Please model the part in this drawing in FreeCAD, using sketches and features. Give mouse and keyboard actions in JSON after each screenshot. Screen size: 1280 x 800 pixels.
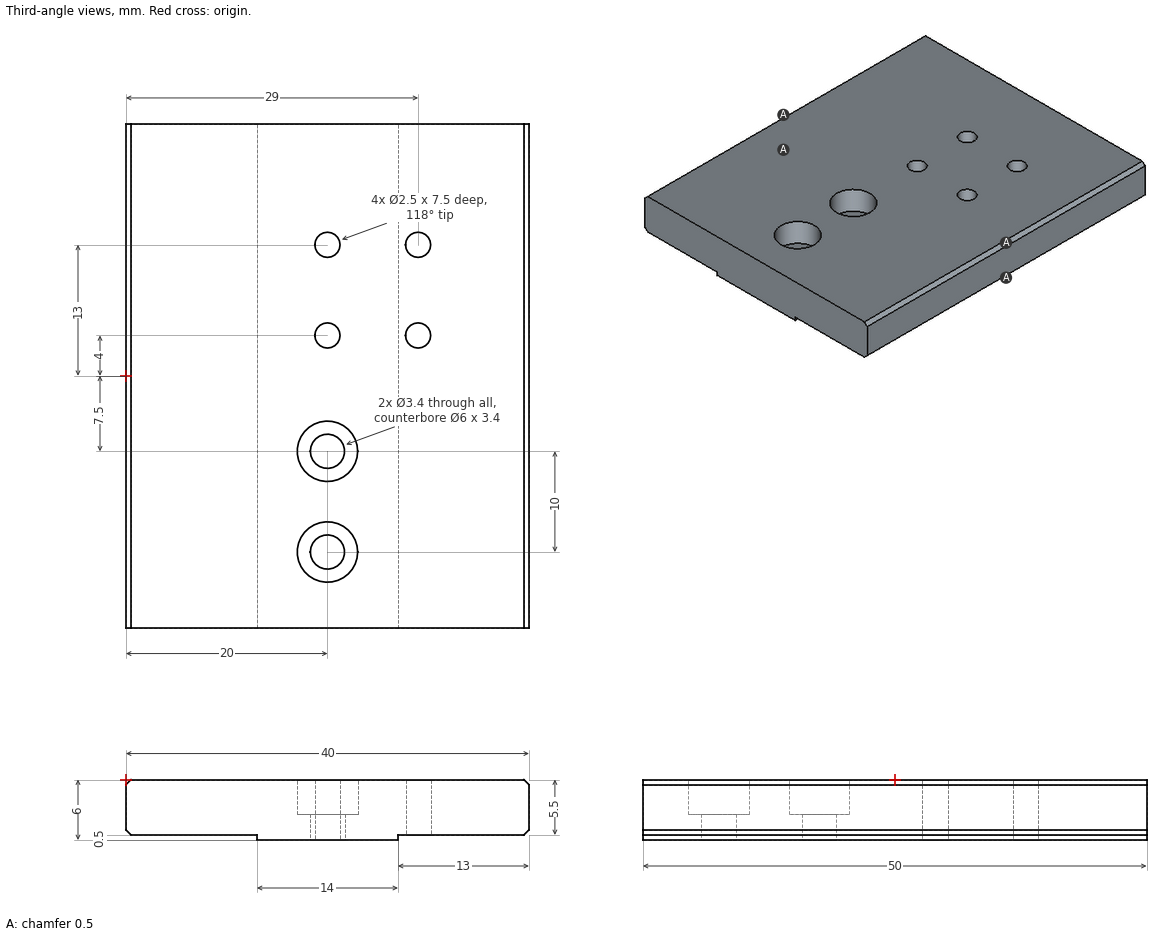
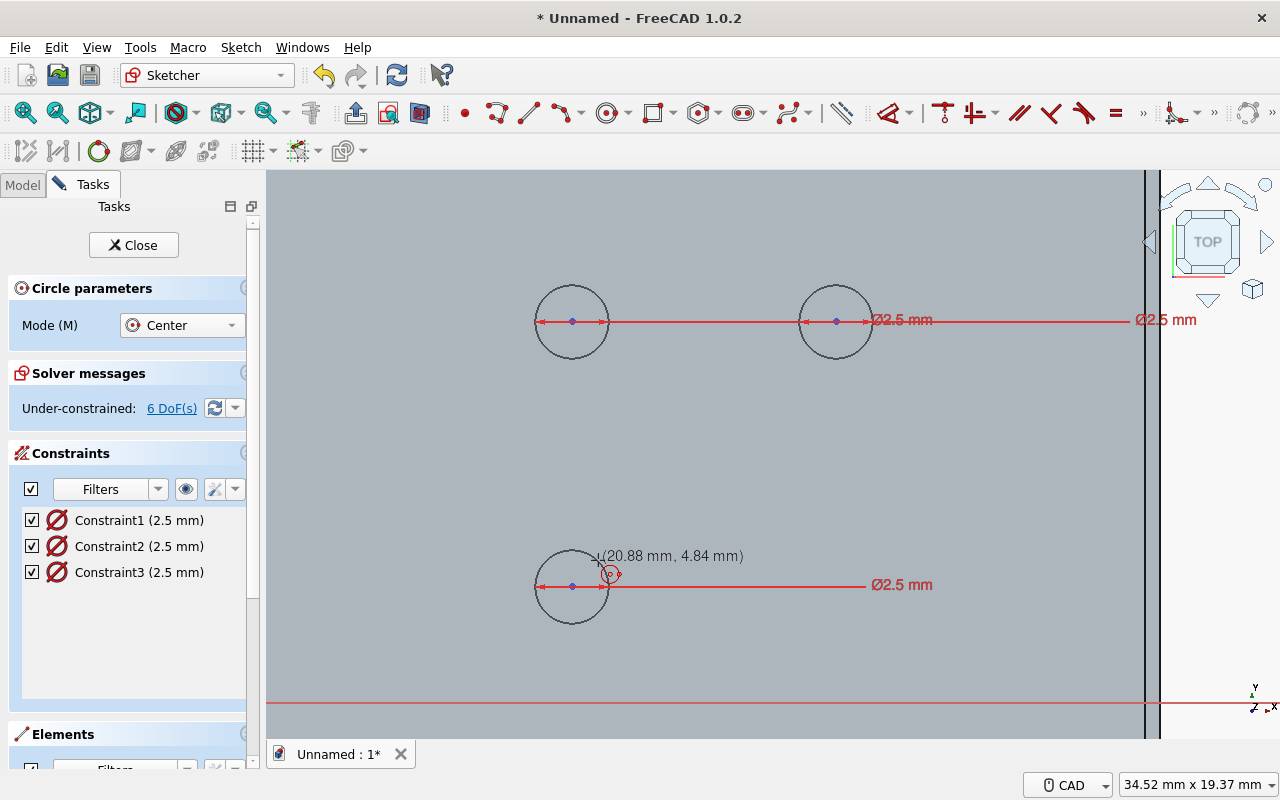
{"action": "left_click", "coordinate": [836, 586]}
{"action": "mouse_move", "coordinate": [862, 560]}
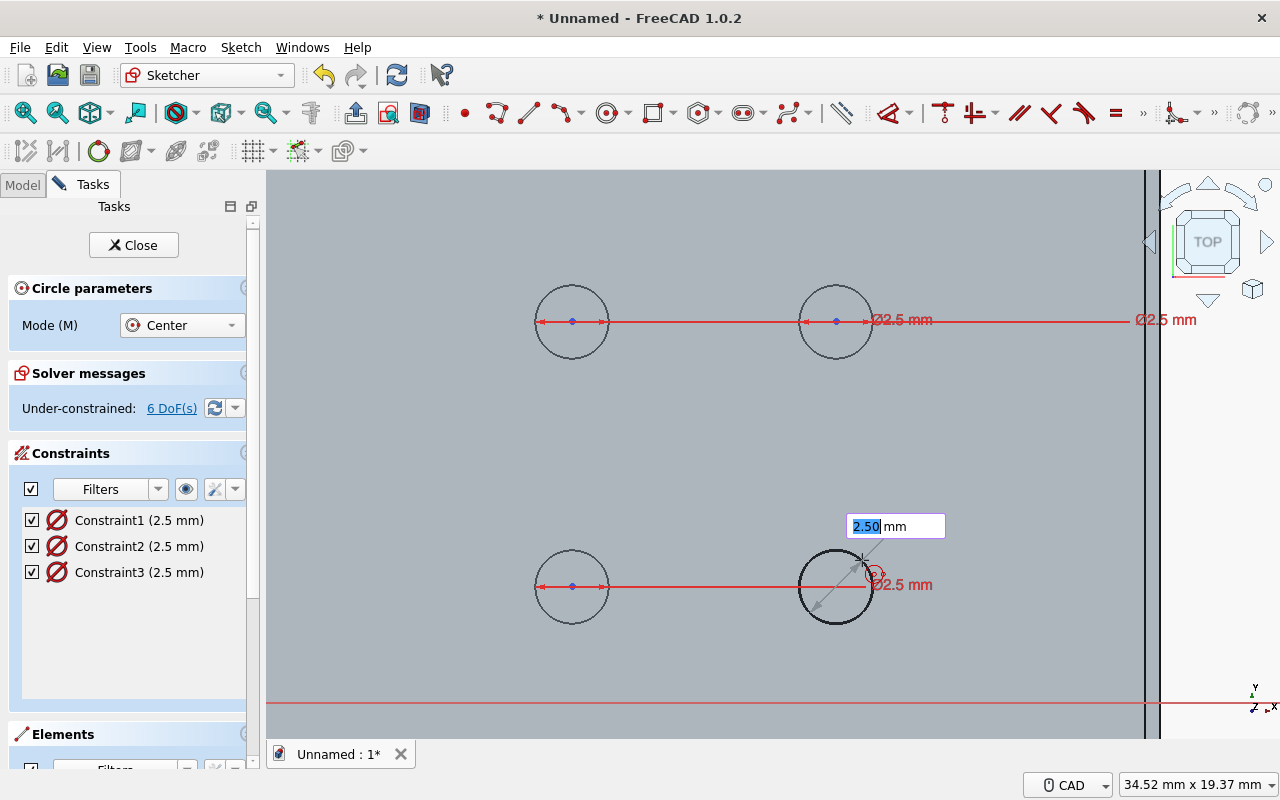
{"action": "type", "text": "2.5"}
{"action": "key", "text": "Return"}
{"action": "key", "text": "Escape"}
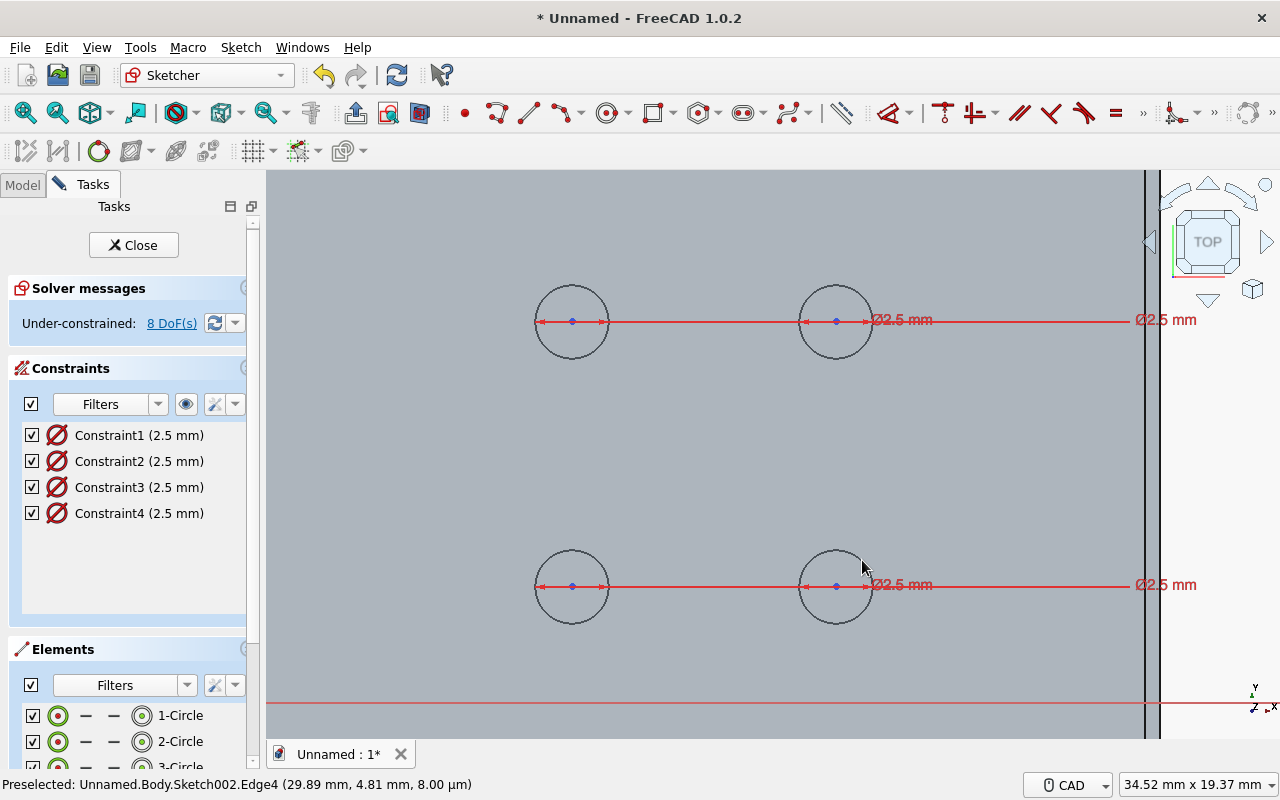
{"action": "left_click", "coordinate": [888, 114]}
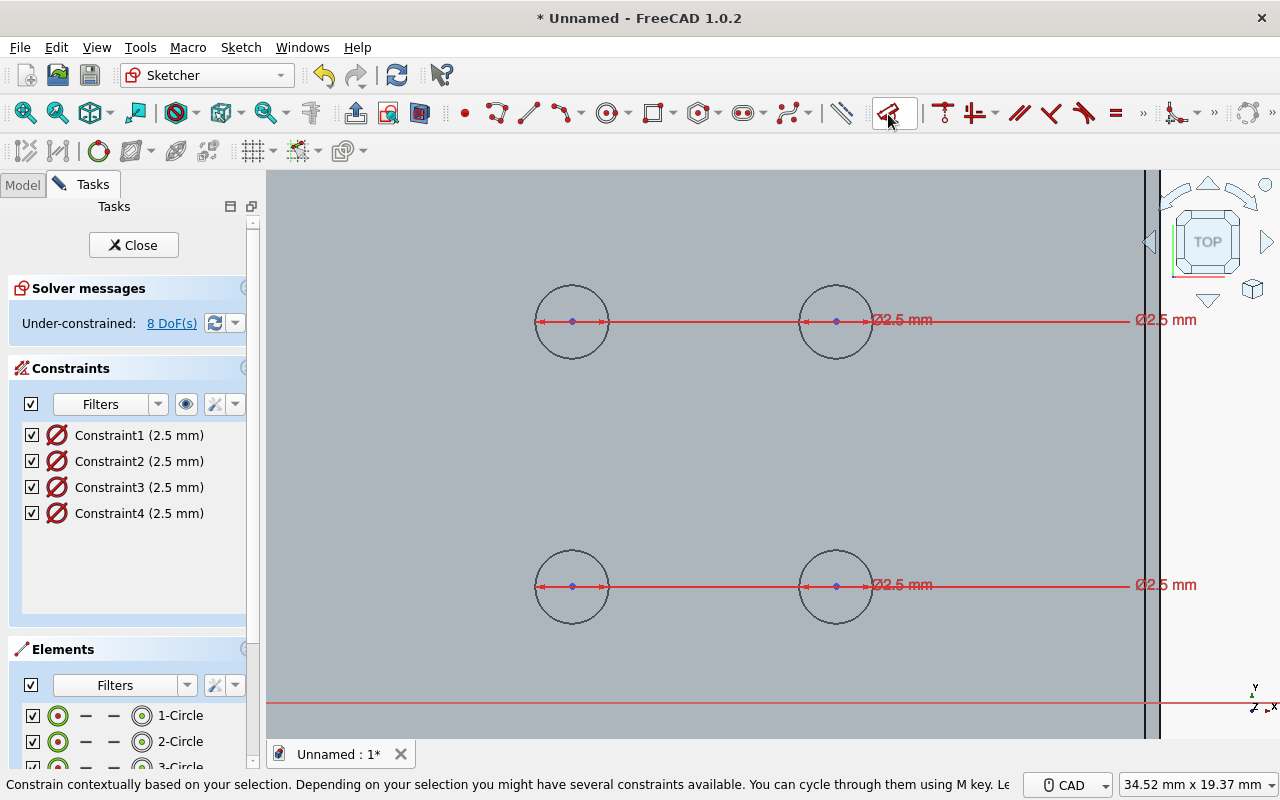
{"action": "left_click", "coordinate": [572, 587]}
{"action": "left_click", "coordinate": [606, 645]}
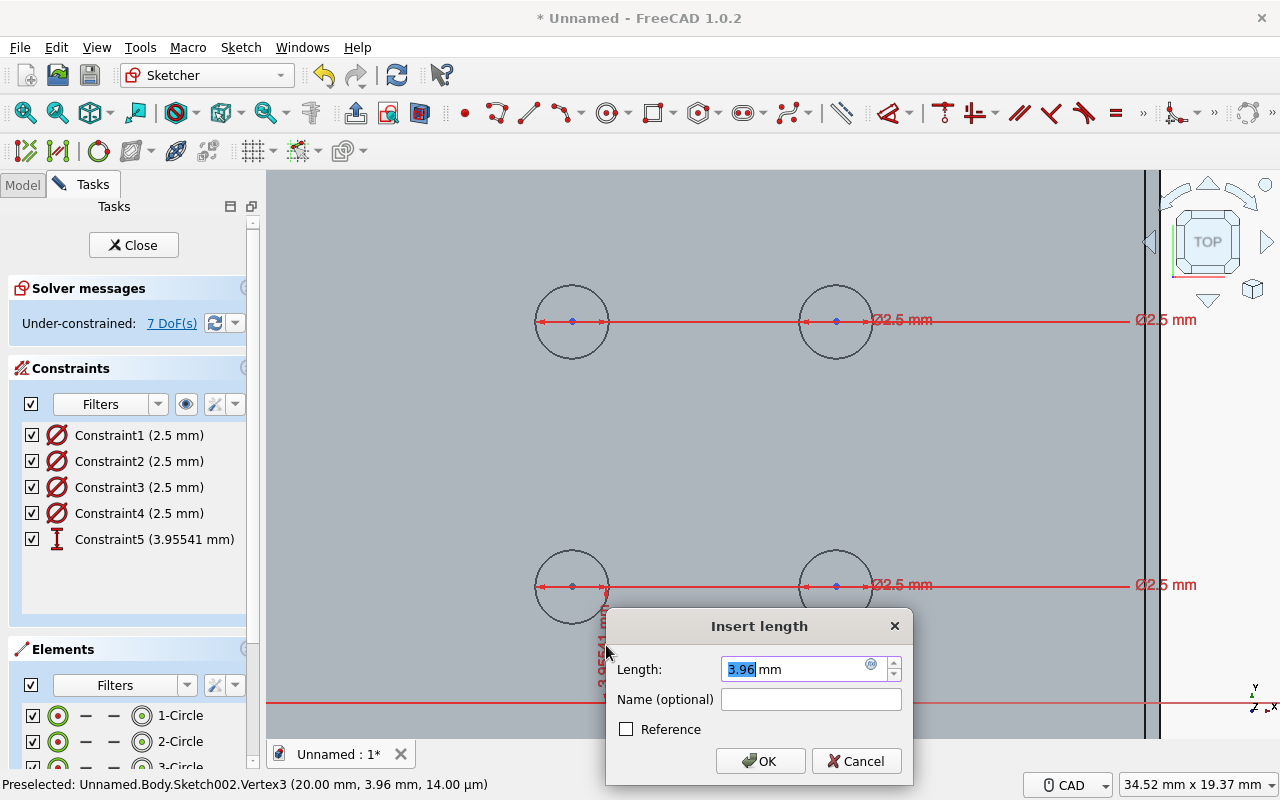
{"action": "type", "text": "4"}
{"action": "key", "text": "Return"}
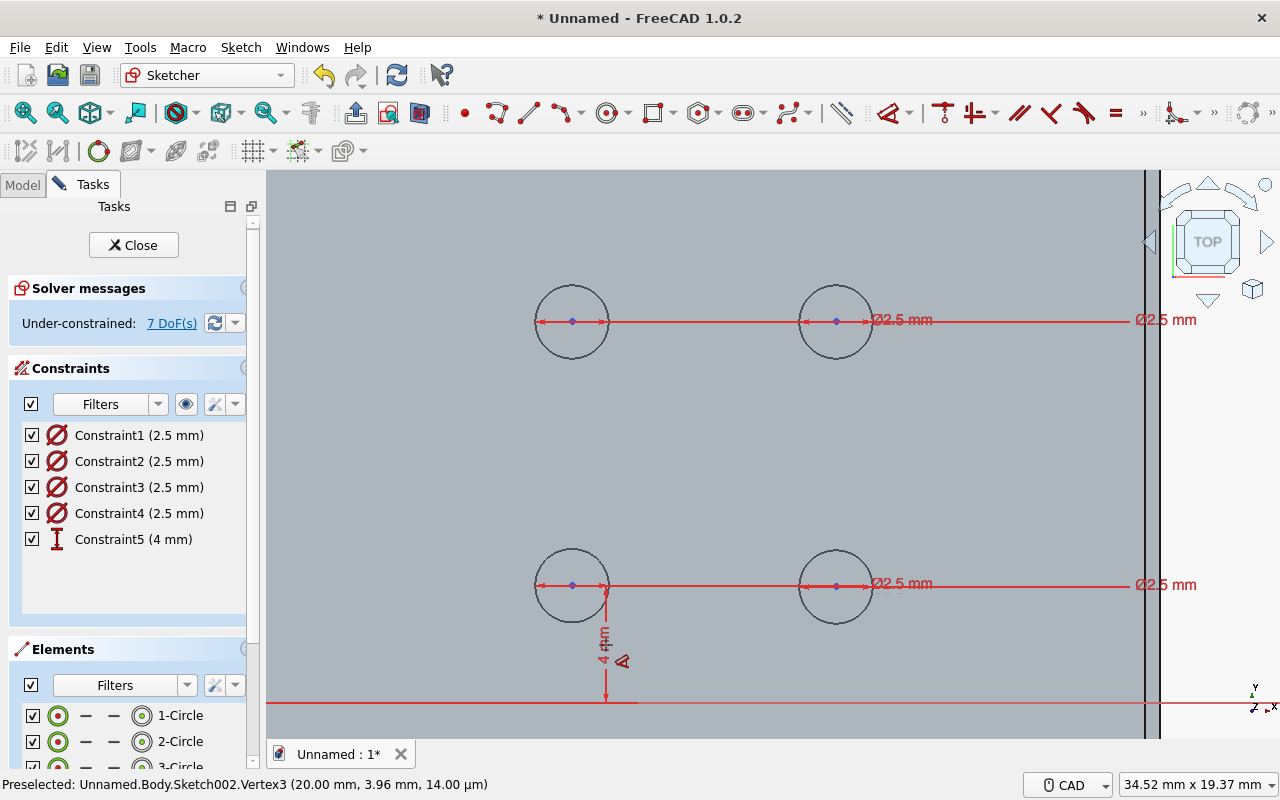
{"action": "left_click", "coordinate": [836, 587]}
{"action": "left_click", "coordinate": [870, 645]}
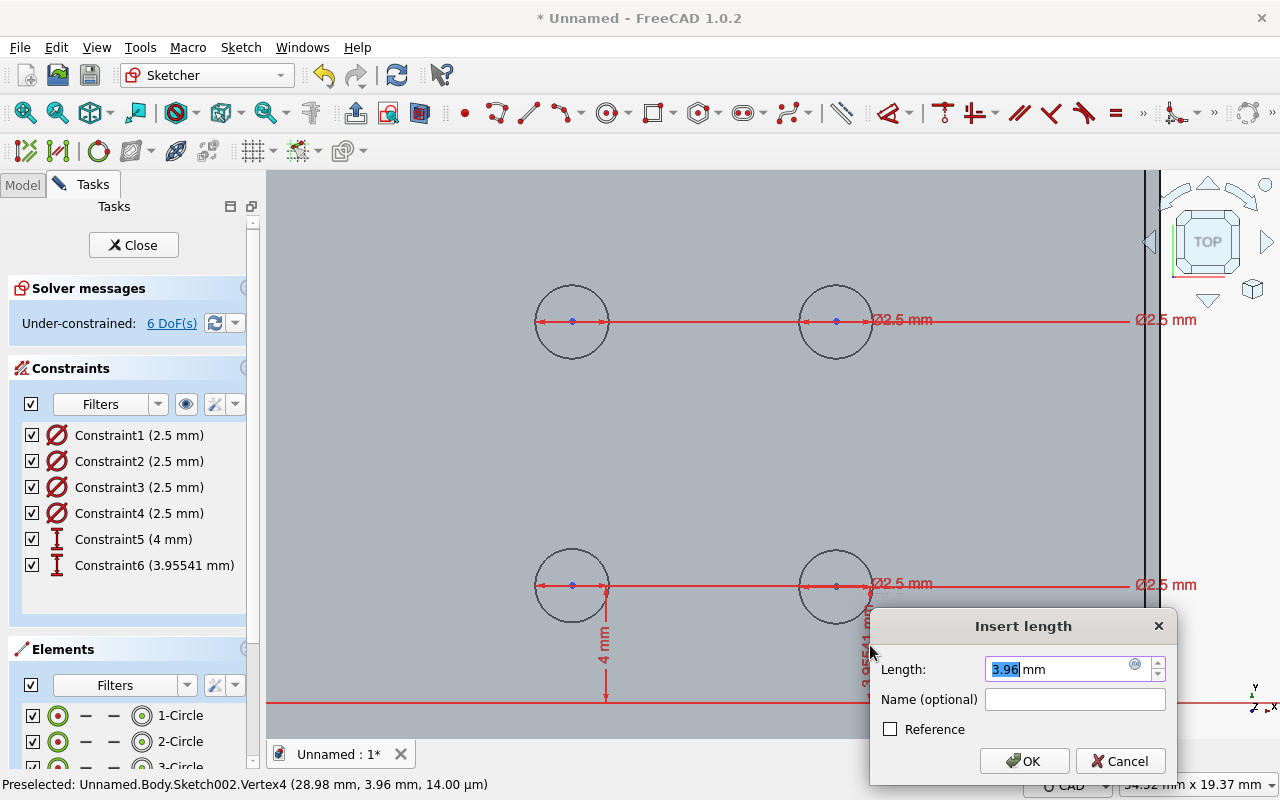
{"action": "type", "text": "4"}
{"action": "key", "text": "Return"}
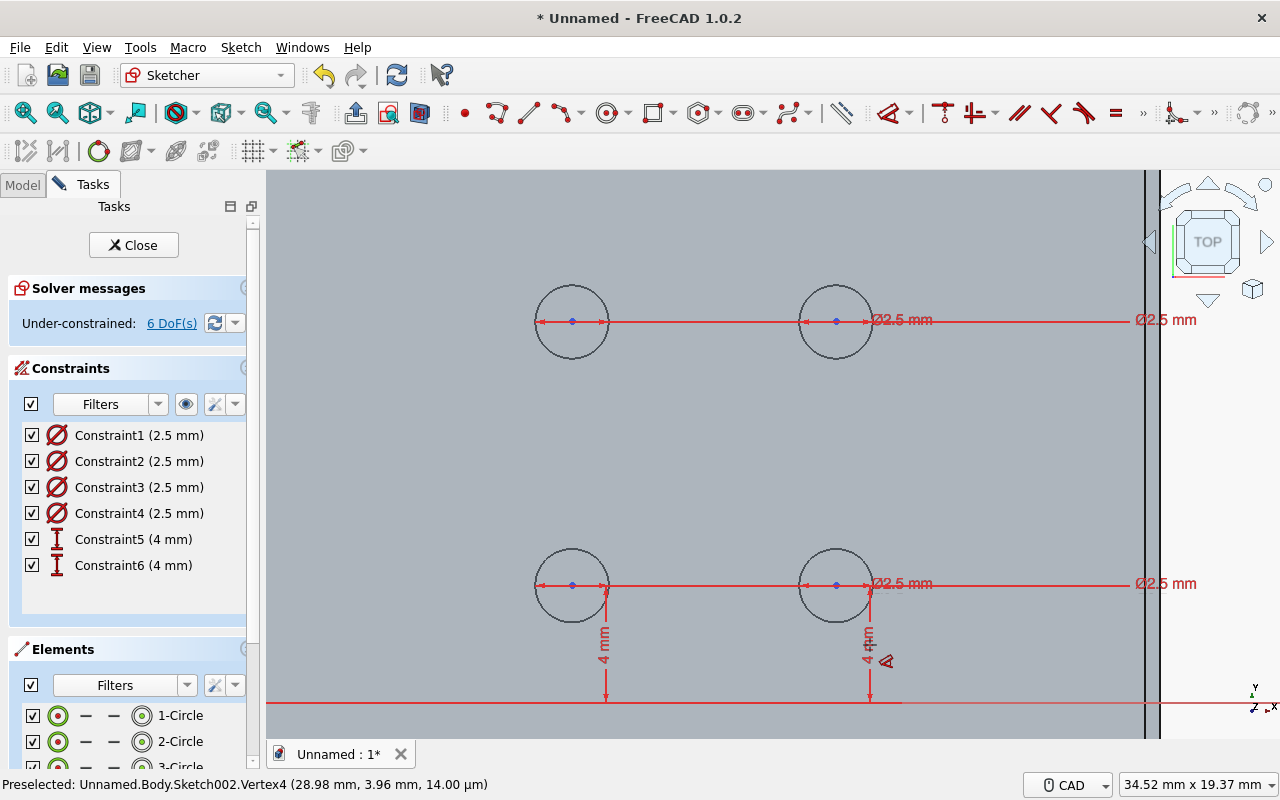
{"action": "left_click", "coordinate": [572, 322]}
{"action": "left_click", "coordinate": [433, 288]}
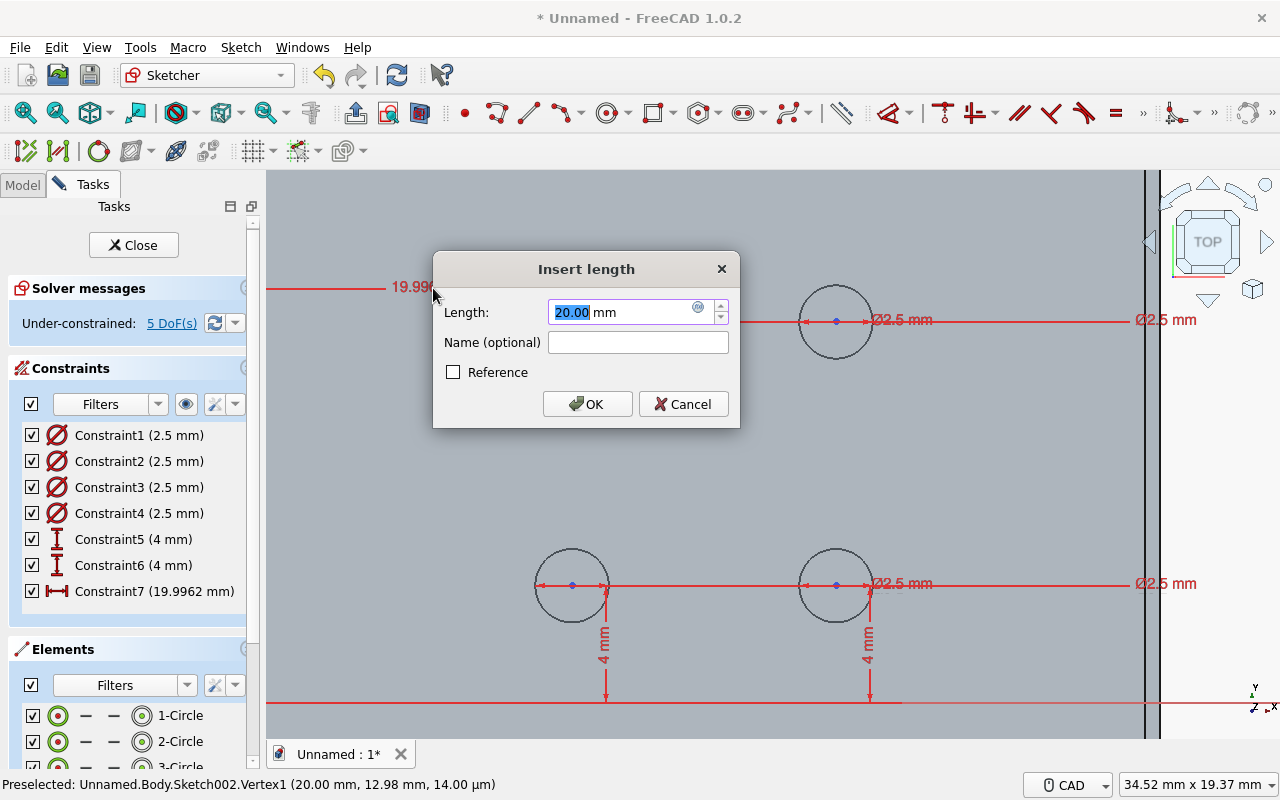
{"action": "type", "text": "20"}
{"action": "key", "text": "Return"}